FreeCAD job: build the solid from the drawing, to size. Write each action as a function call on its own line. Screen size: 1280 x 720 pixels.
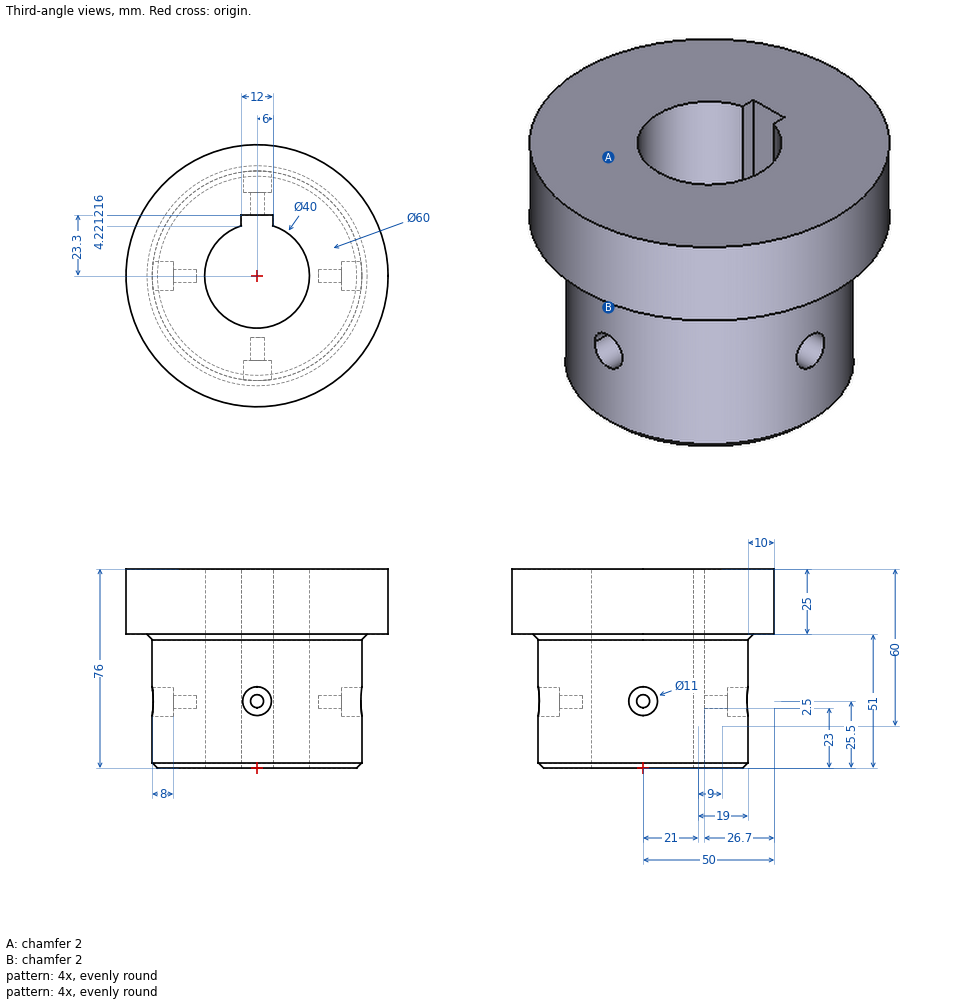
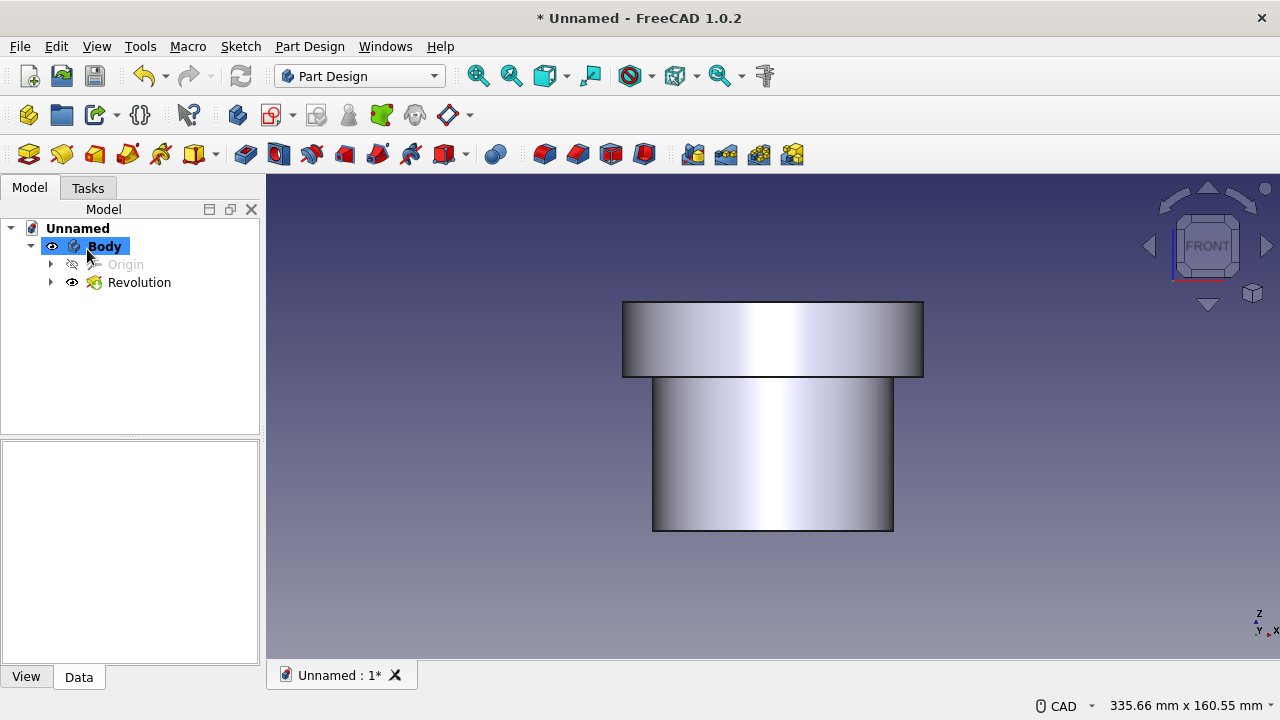
key(3)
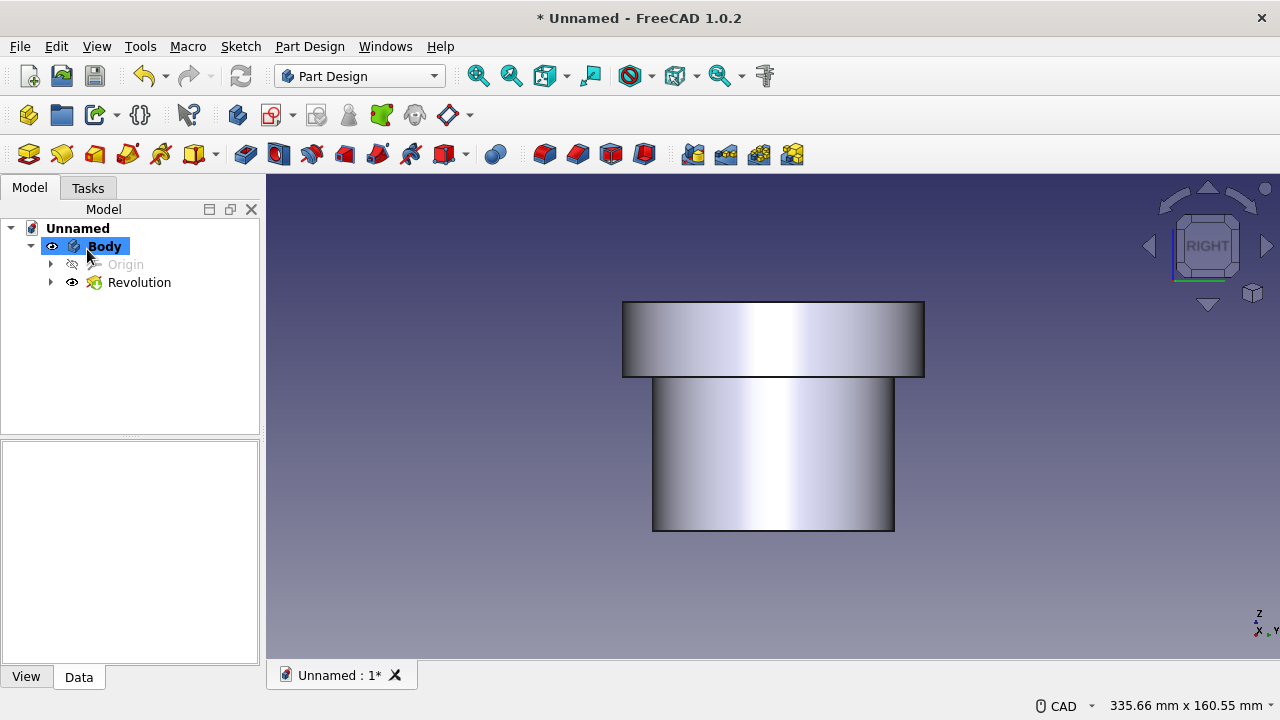
key(5)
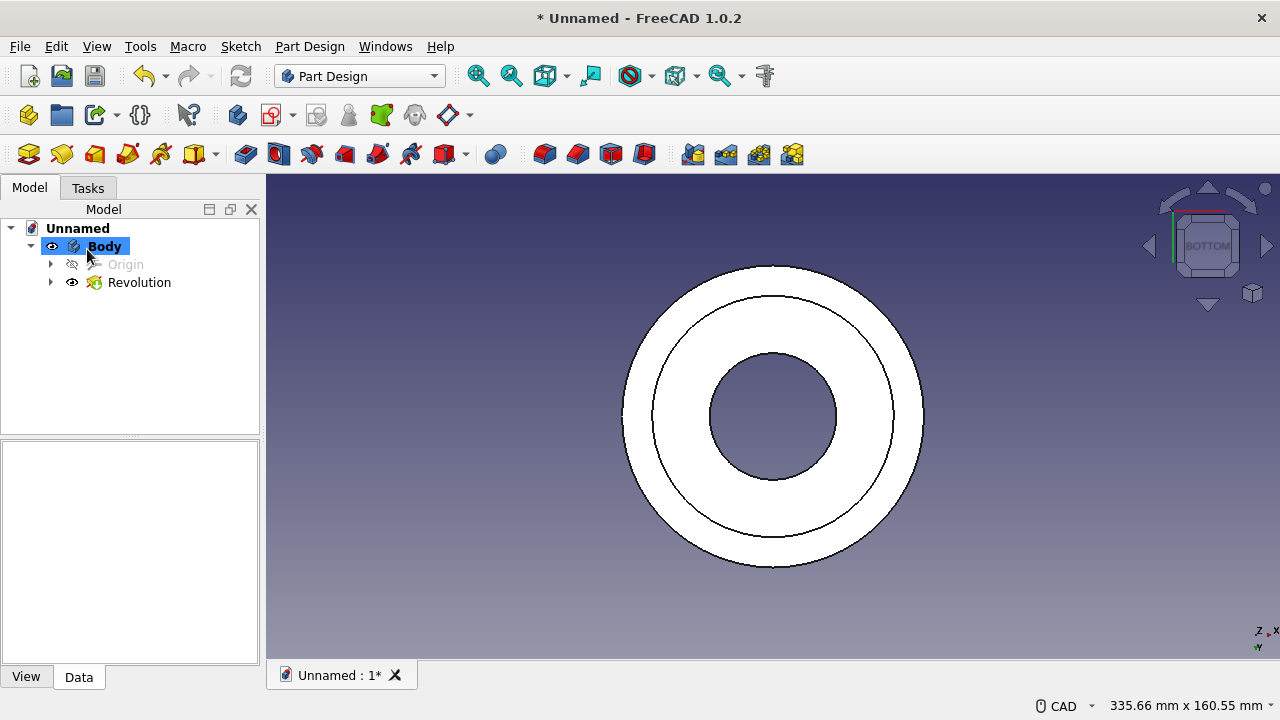
key(4)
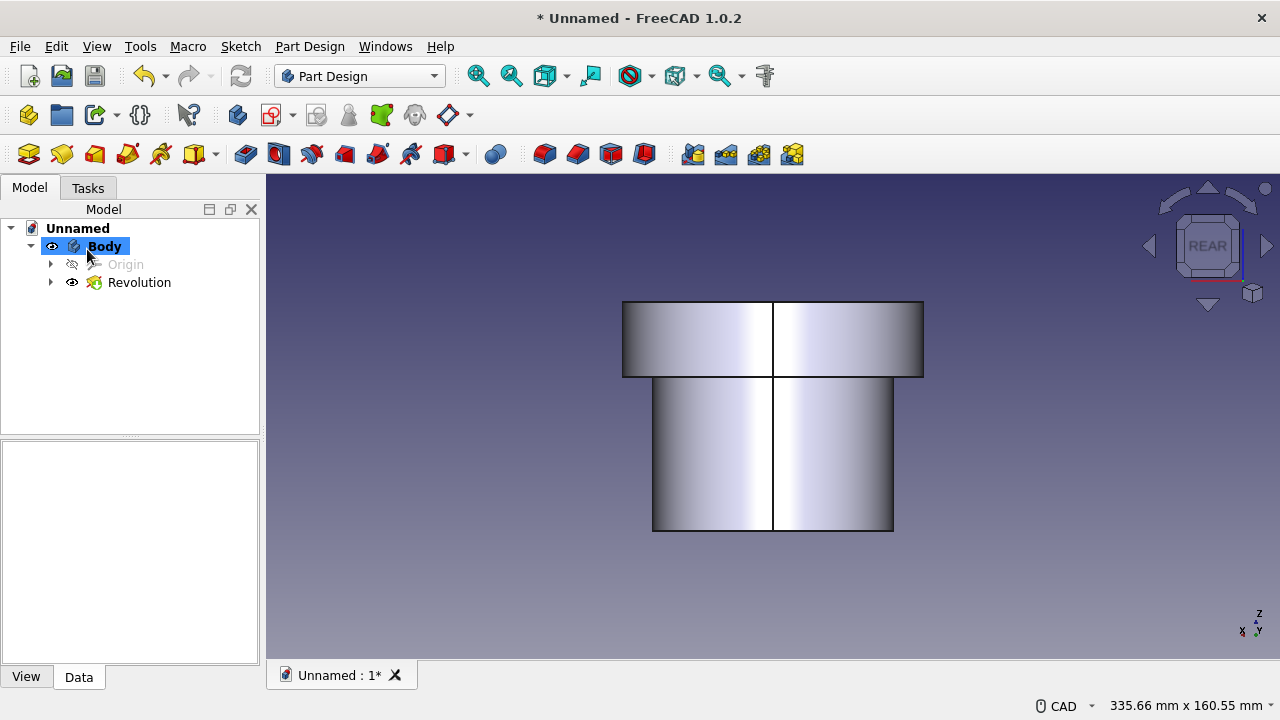
key(6)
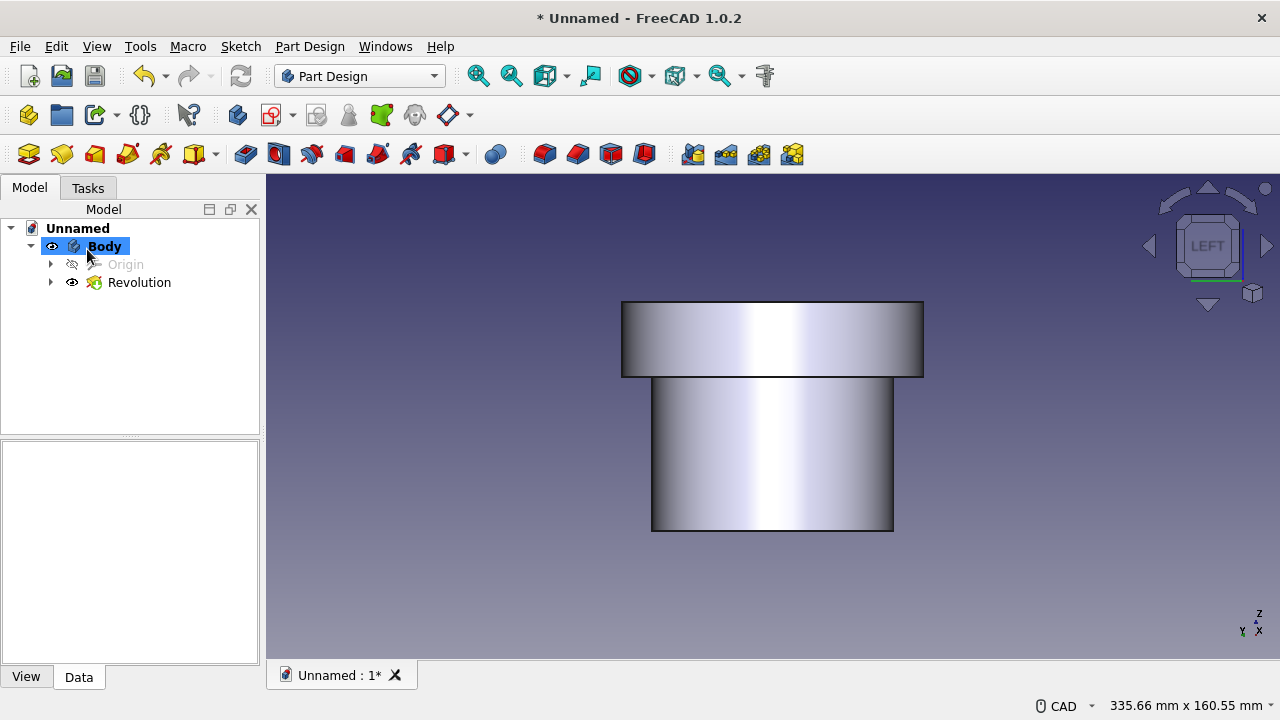
key(v)
key(3)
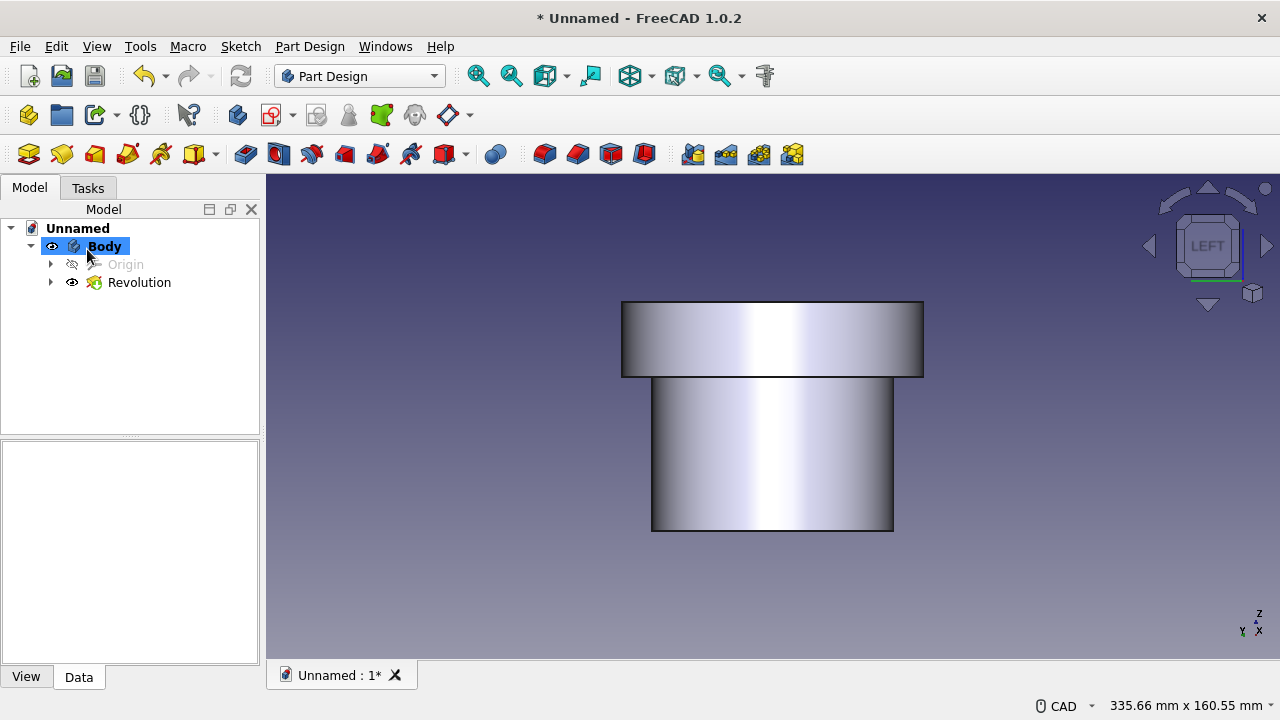
key(0)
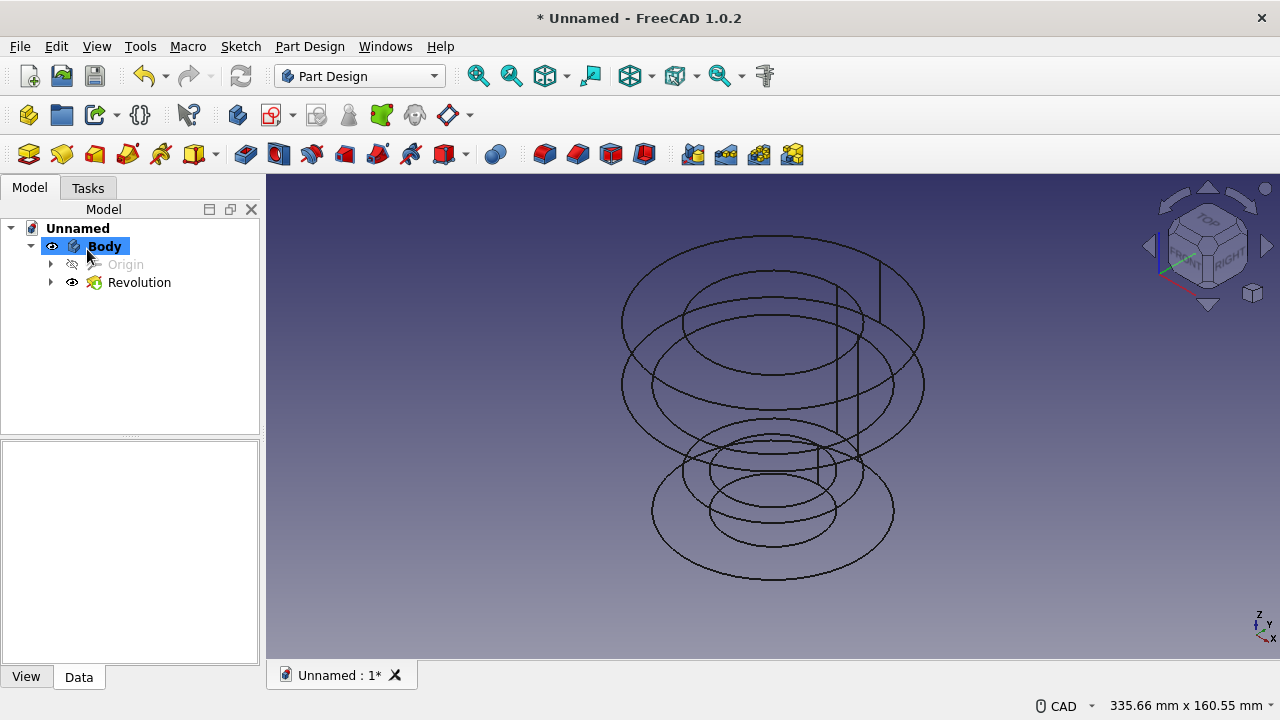
click(688, 433)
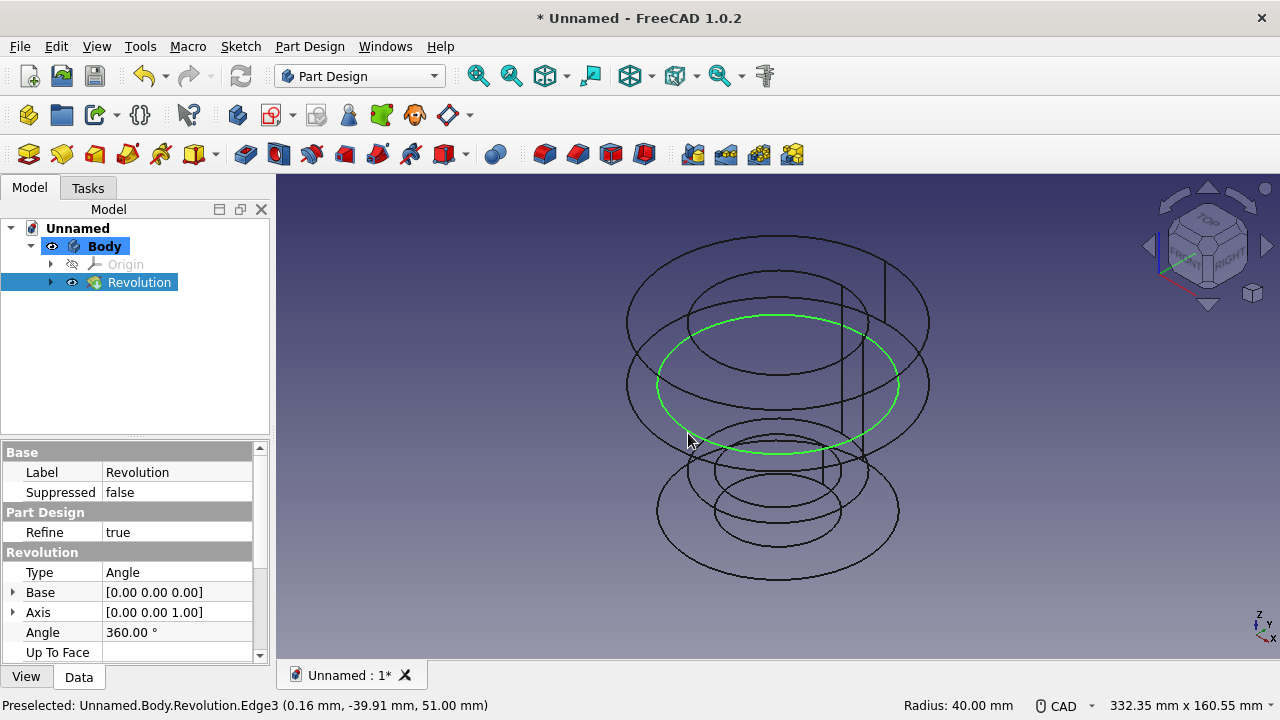
key(v)
key(1)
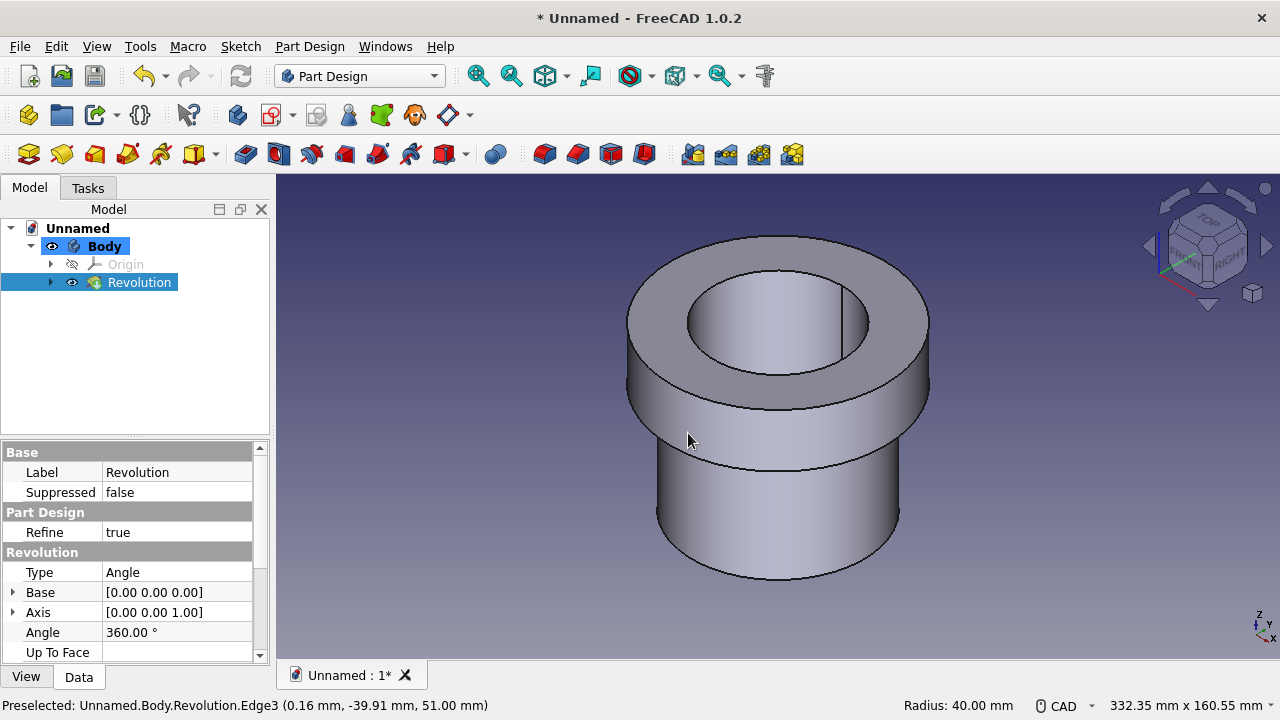
click(578, 154)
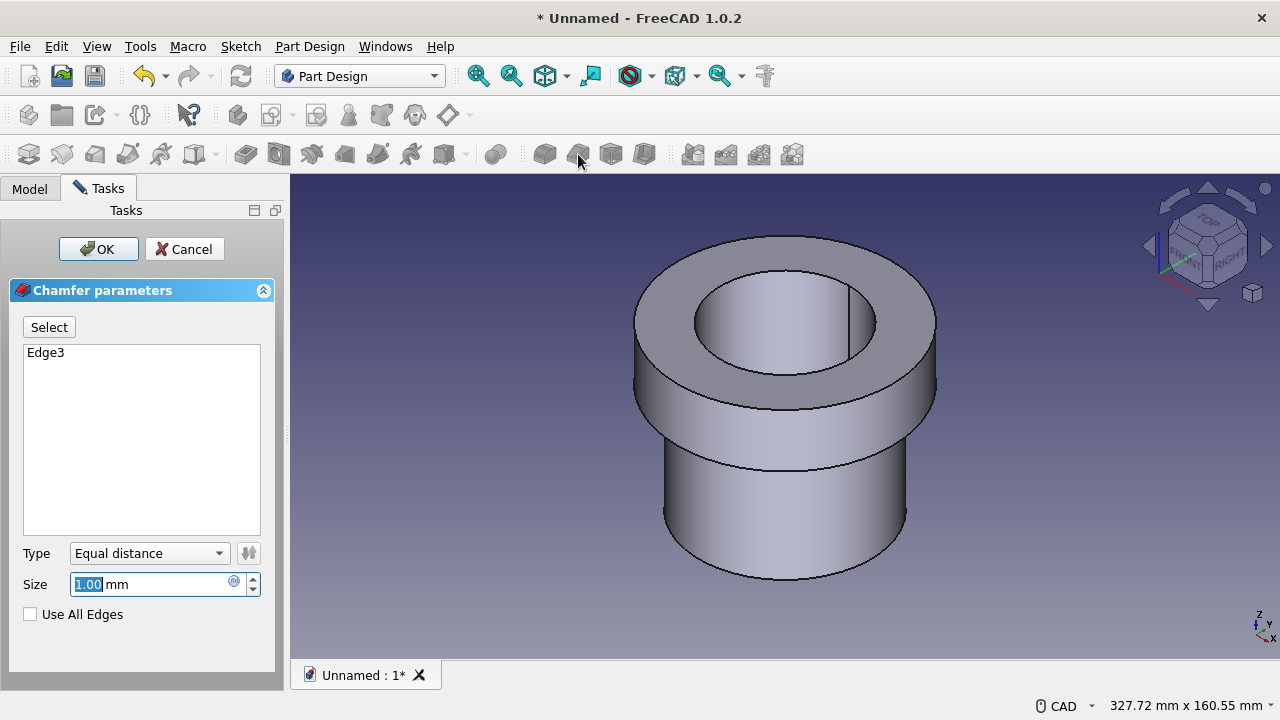
text(2)
key(Tab)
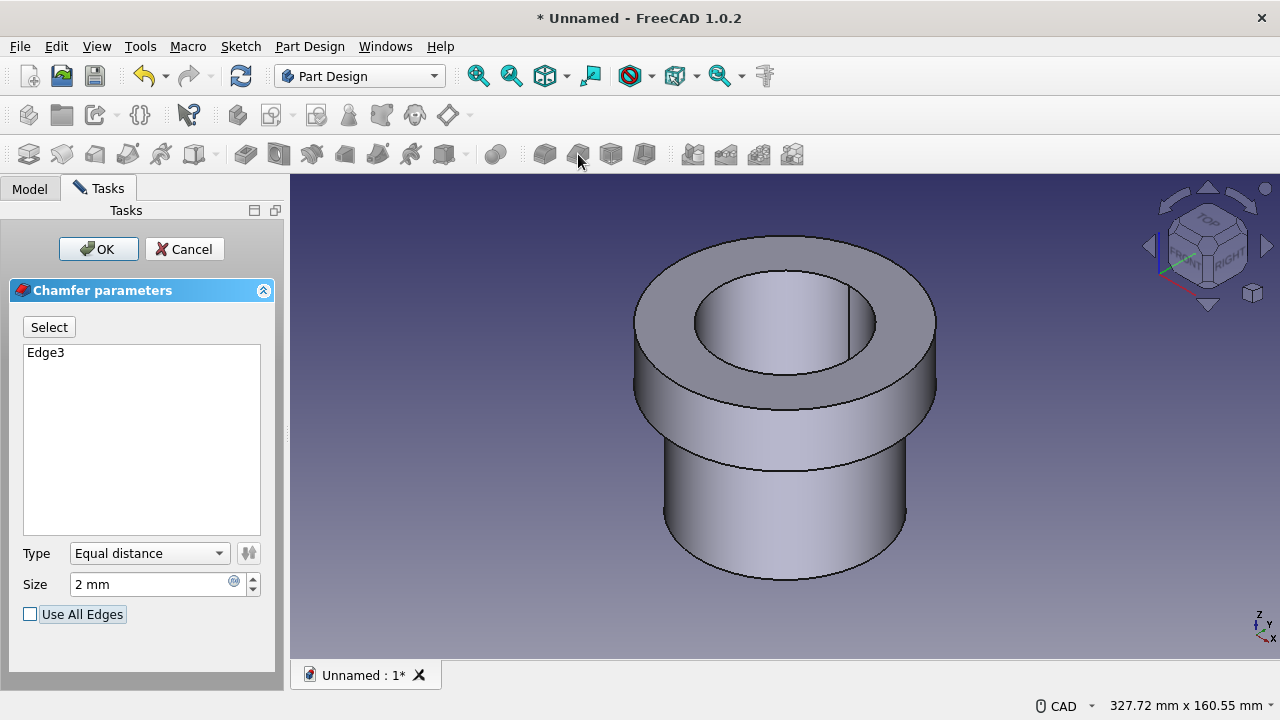
click(99, 249)